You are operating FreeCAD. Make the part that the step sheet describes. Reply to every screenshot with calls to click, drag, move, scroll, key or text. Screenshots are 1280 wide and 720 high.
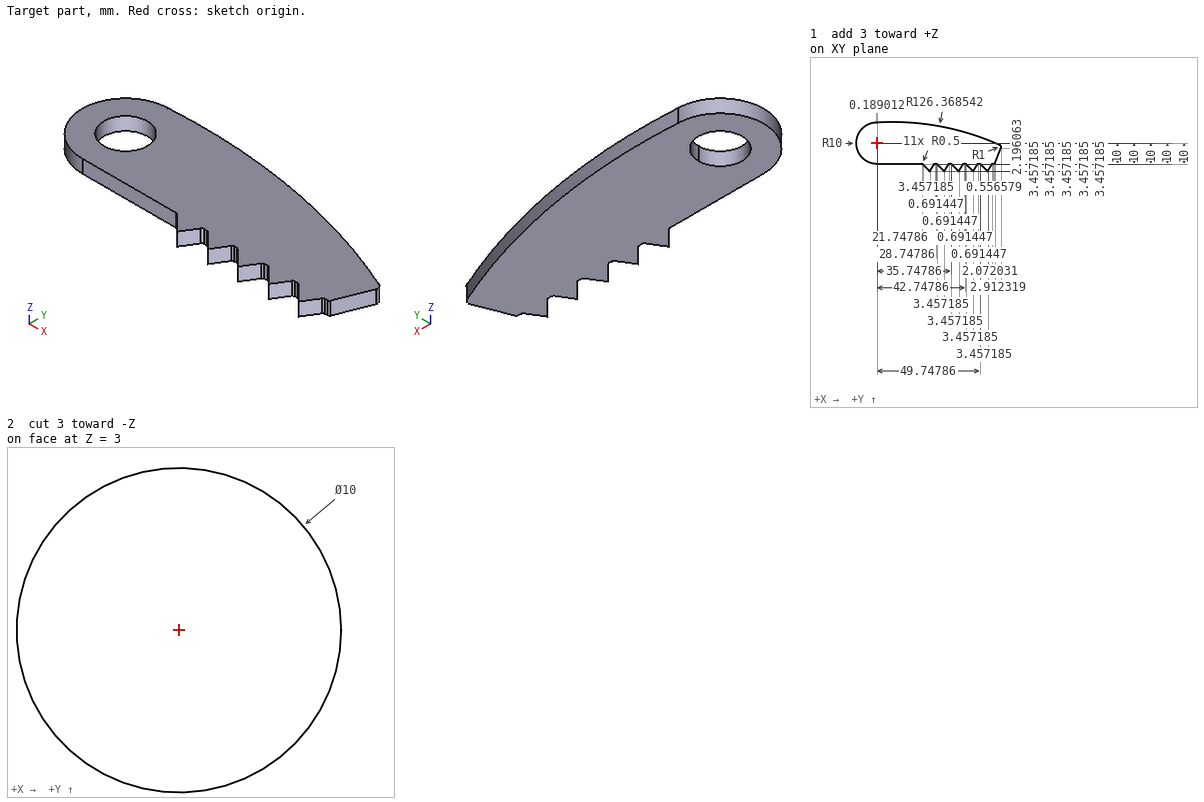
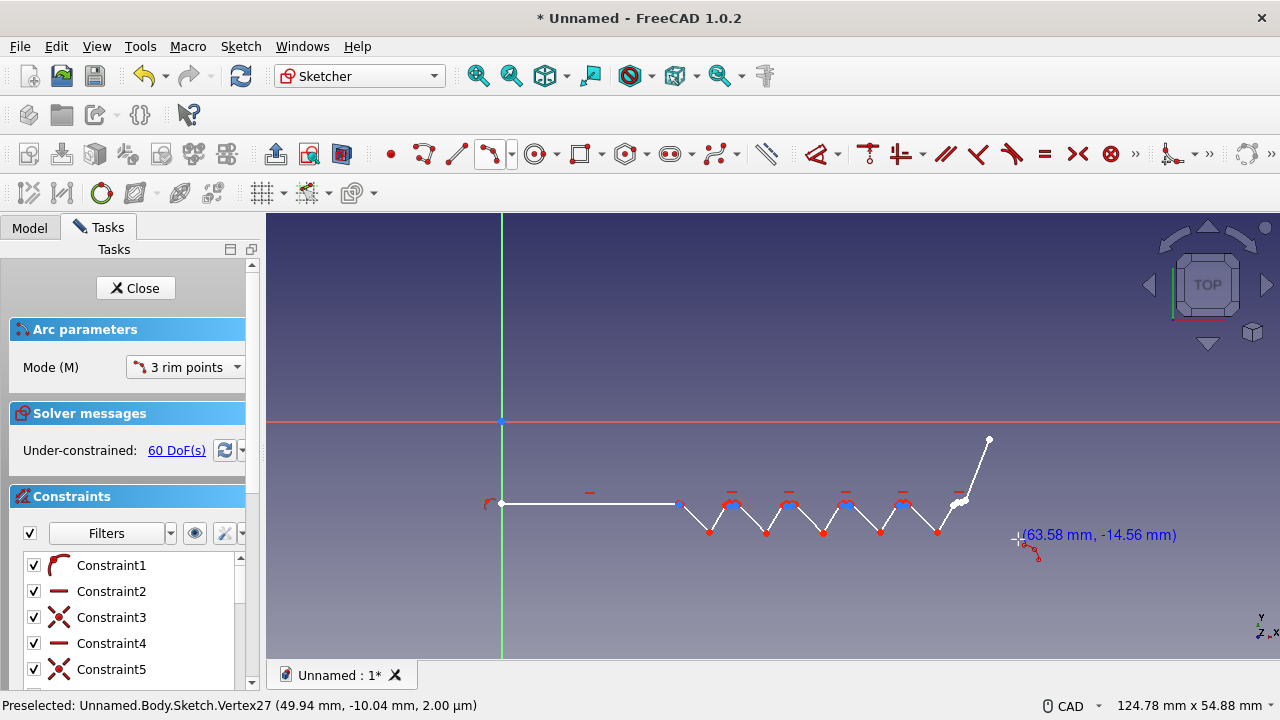
scroll(954, 505, up, 7)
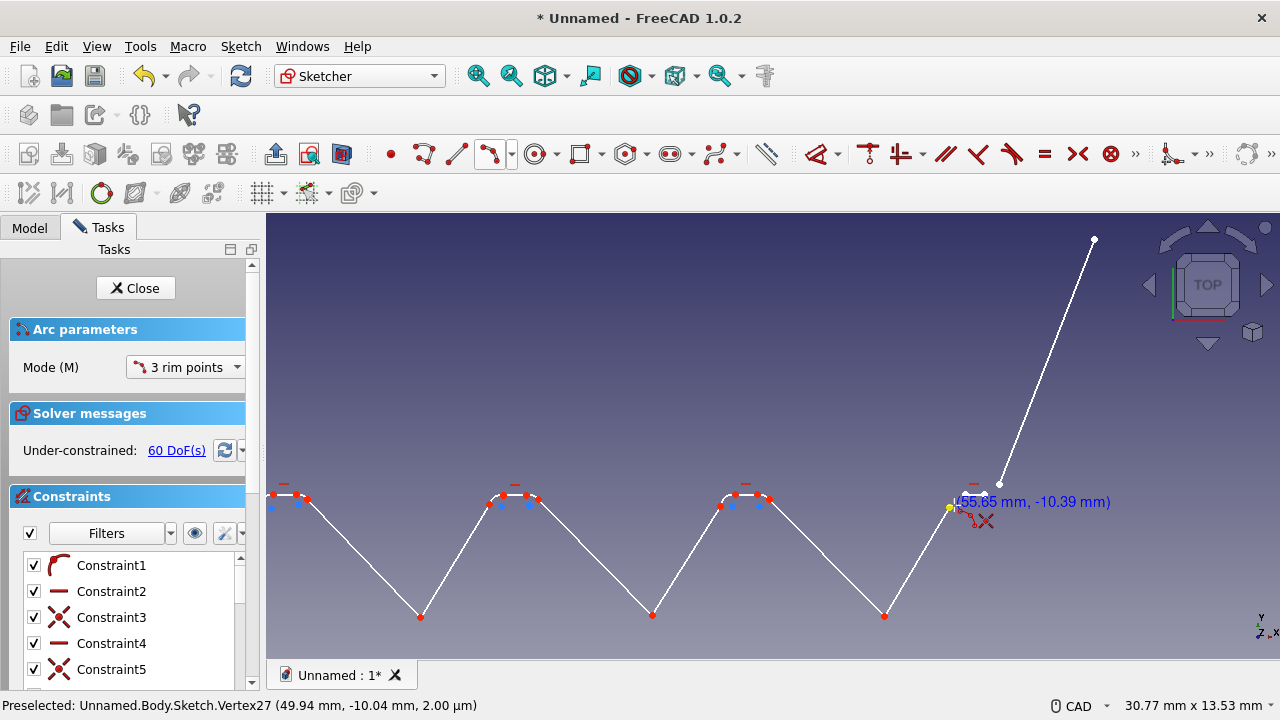
click(950, 507)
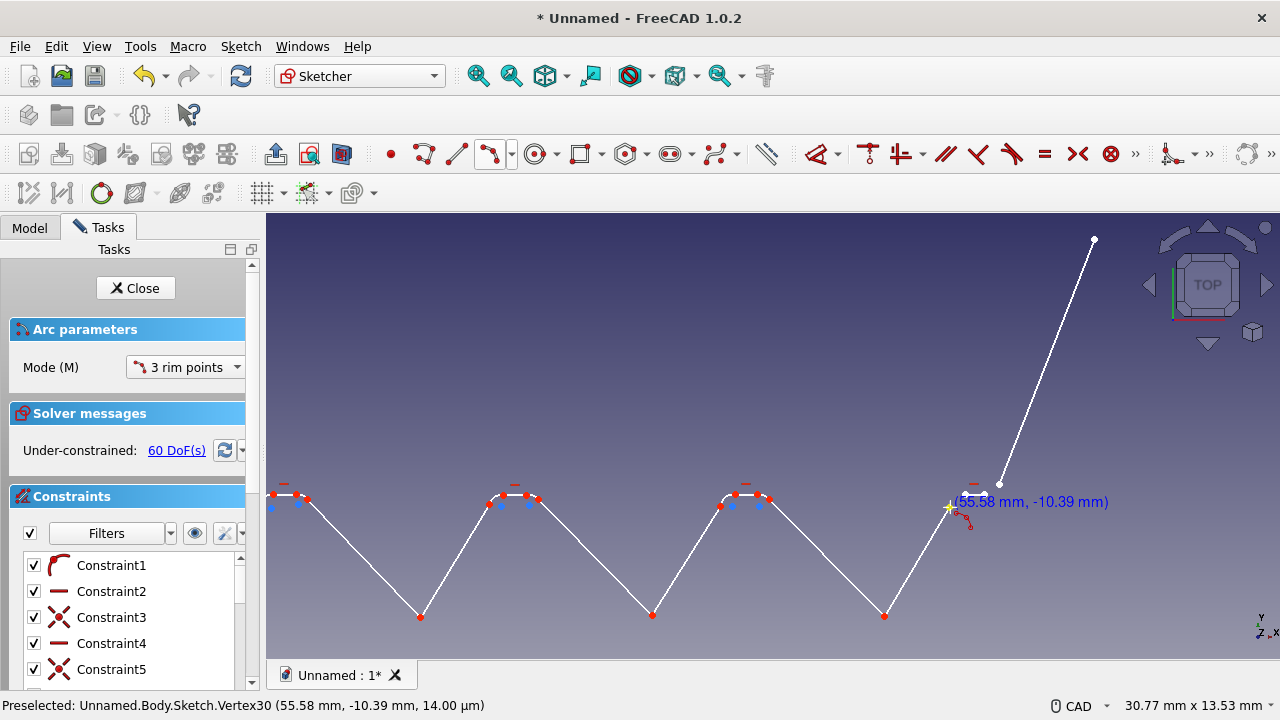
scroll(965, 494, up, 3)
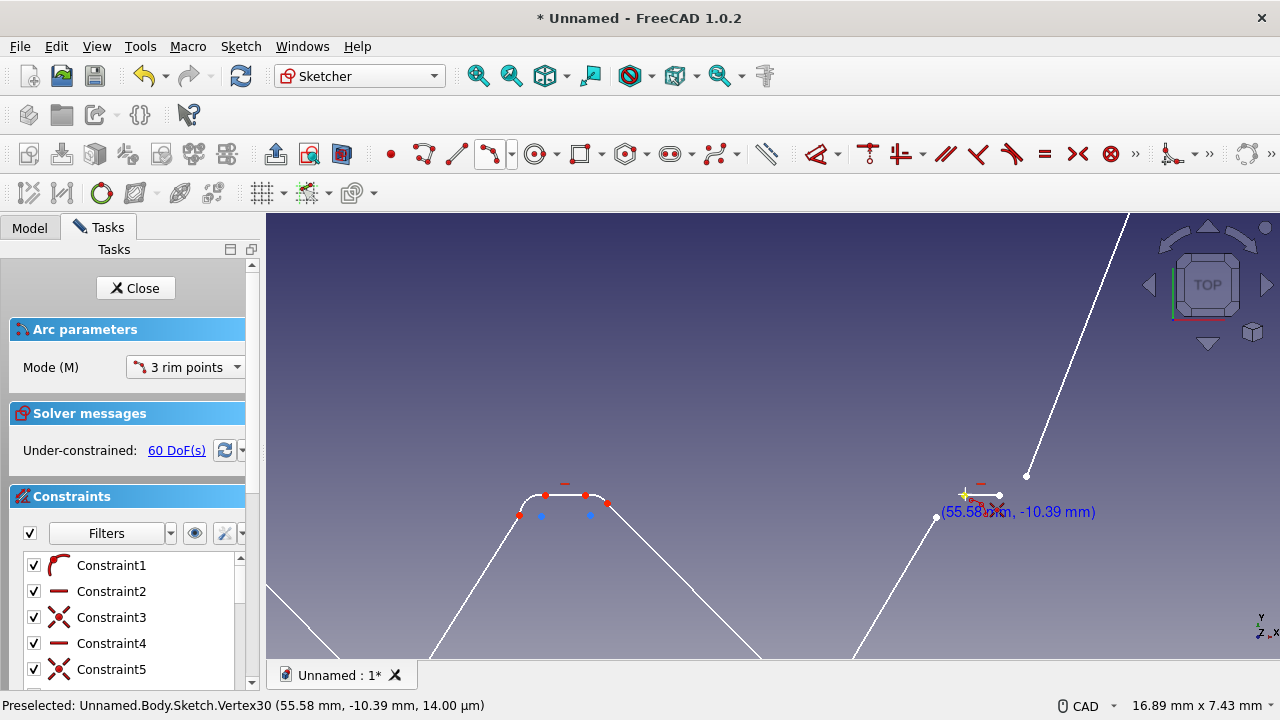
click(965, 495)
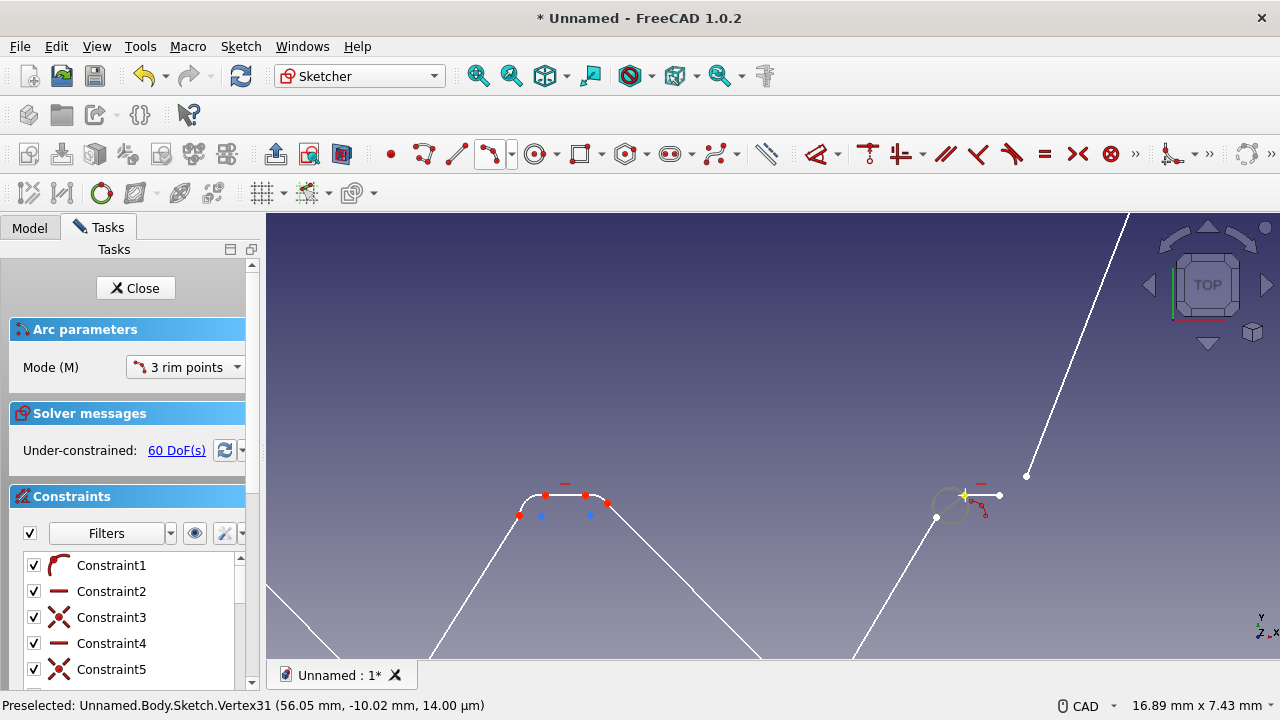
scroll(951, 497, up, 8)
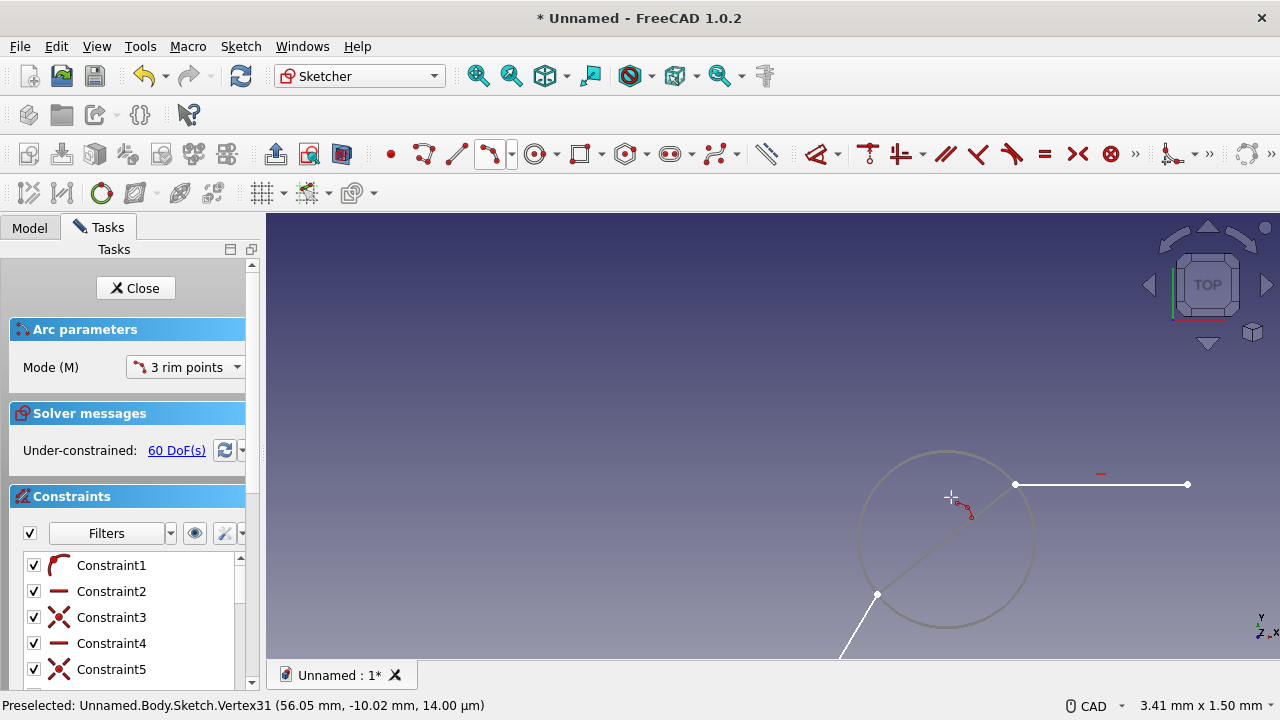
click(946, 496)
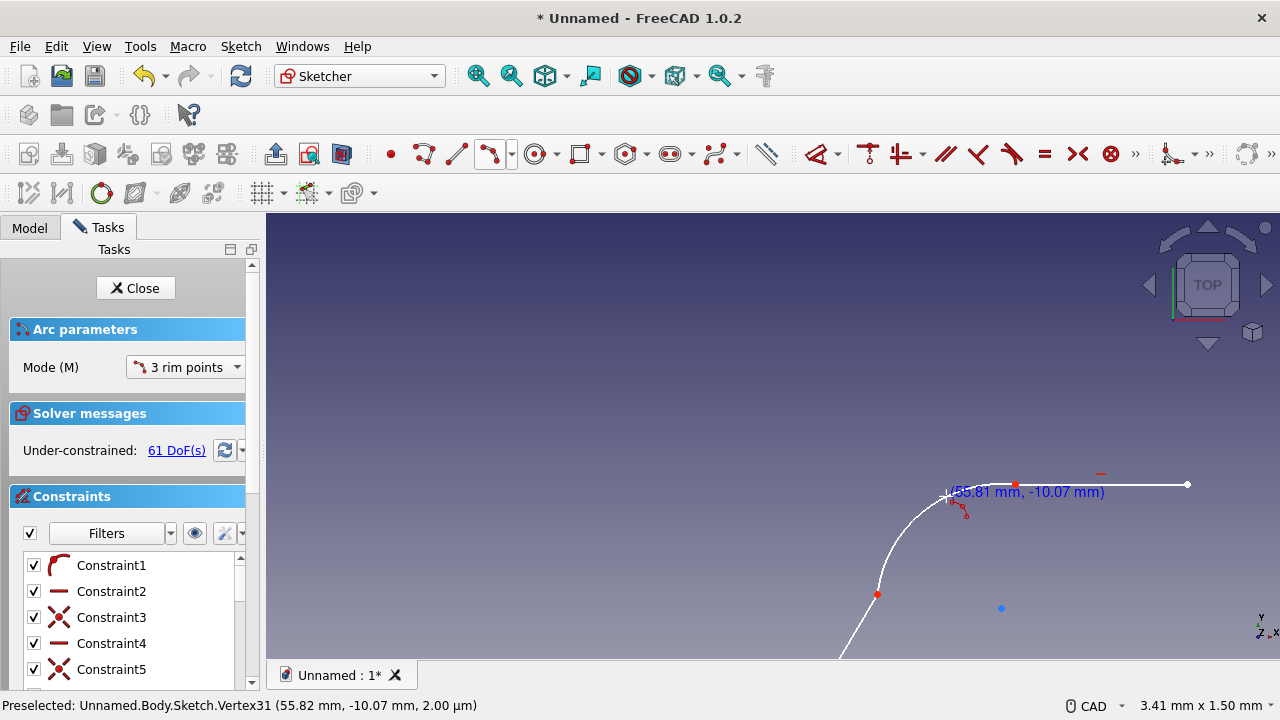
scroll(1013, 519, down, 17)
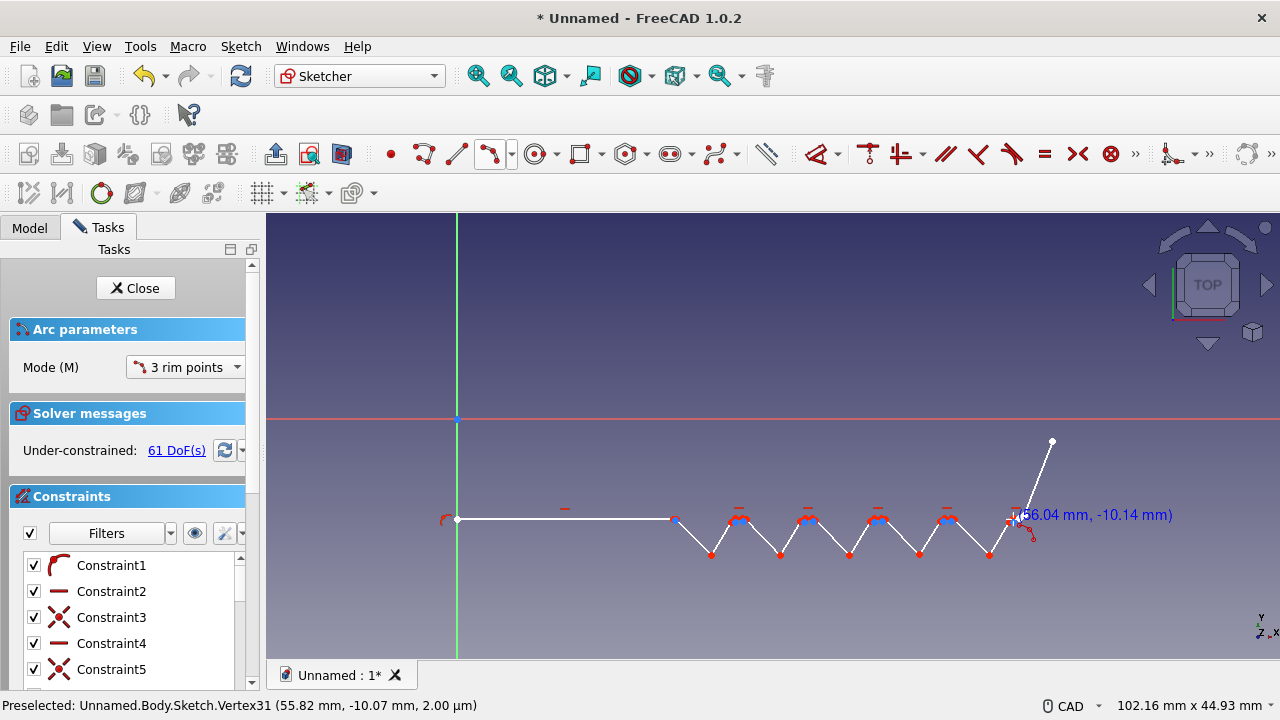
scroll(1019, 518, up, 9)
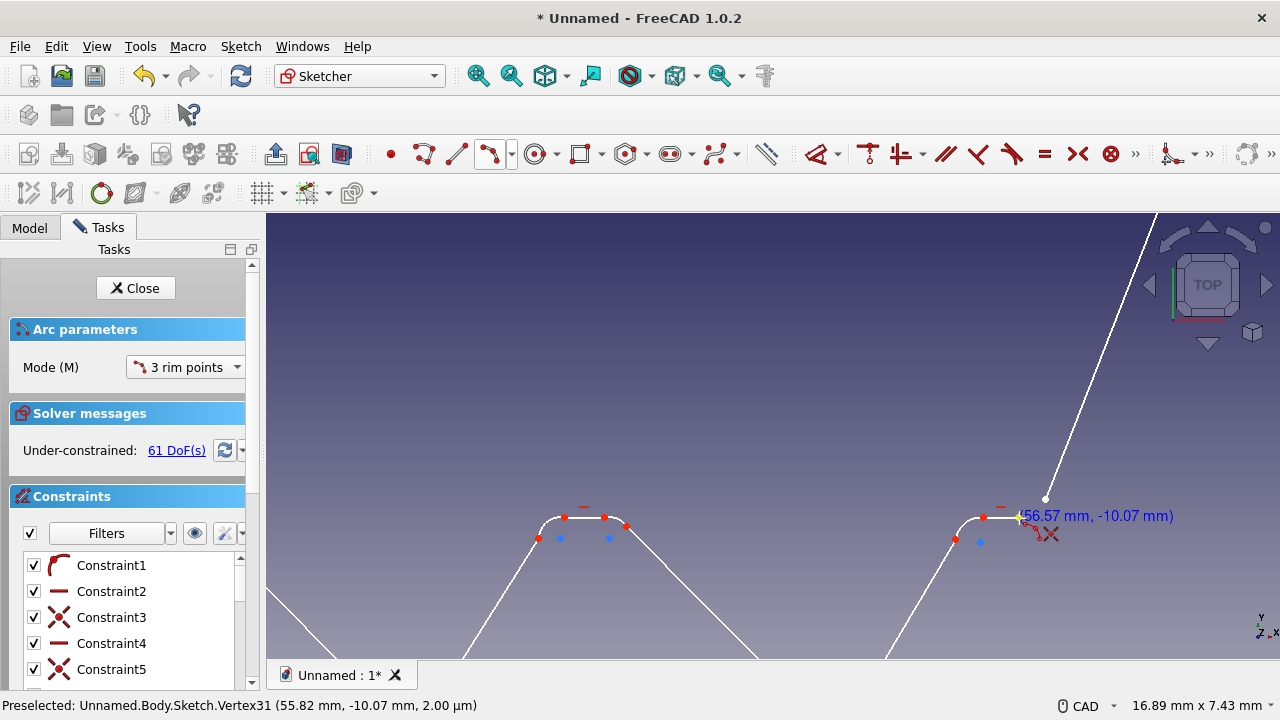
click(1018, 518)
click(1046, 499)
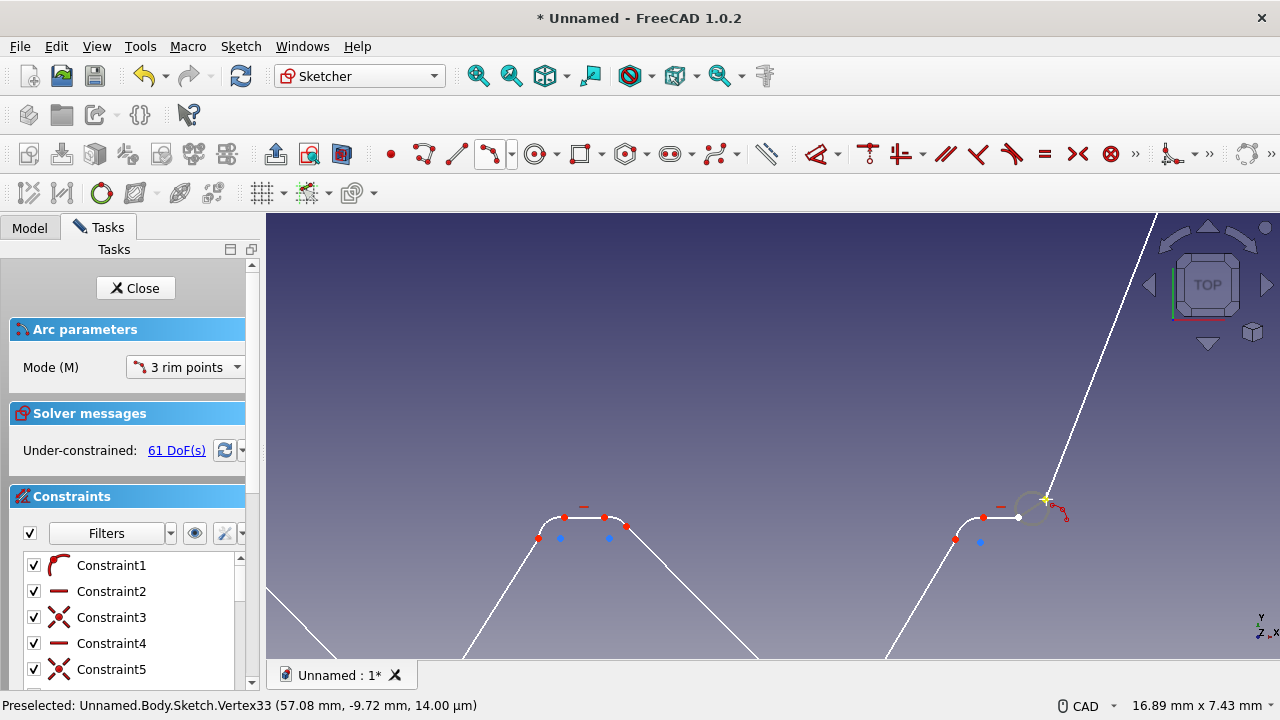
scroll(1035, 511, up, 6)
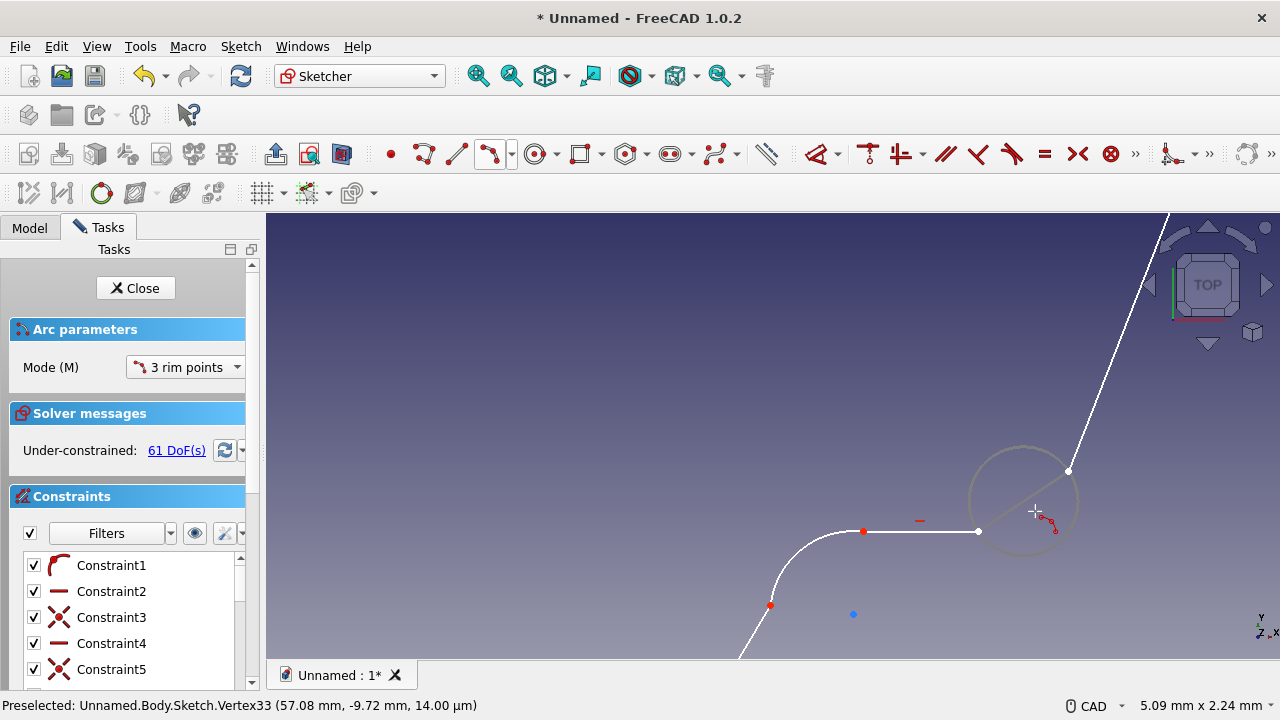
click(1032, 509)